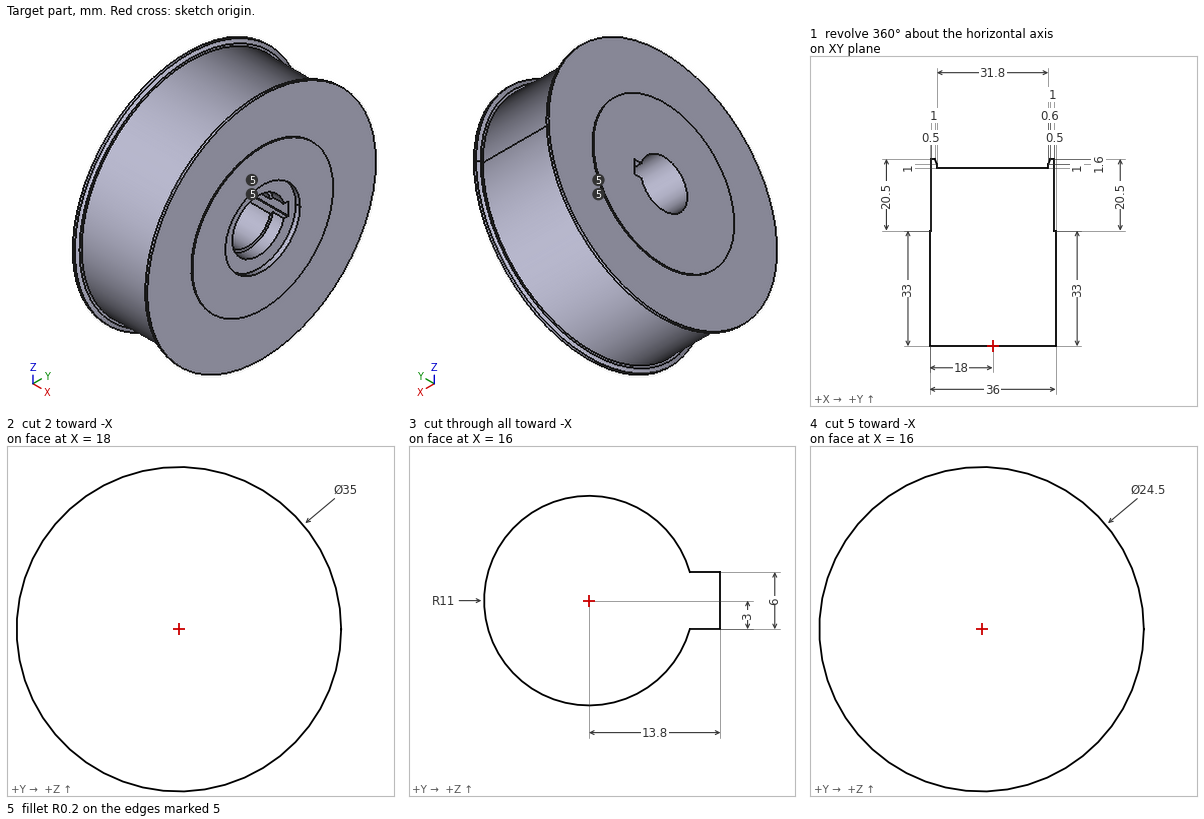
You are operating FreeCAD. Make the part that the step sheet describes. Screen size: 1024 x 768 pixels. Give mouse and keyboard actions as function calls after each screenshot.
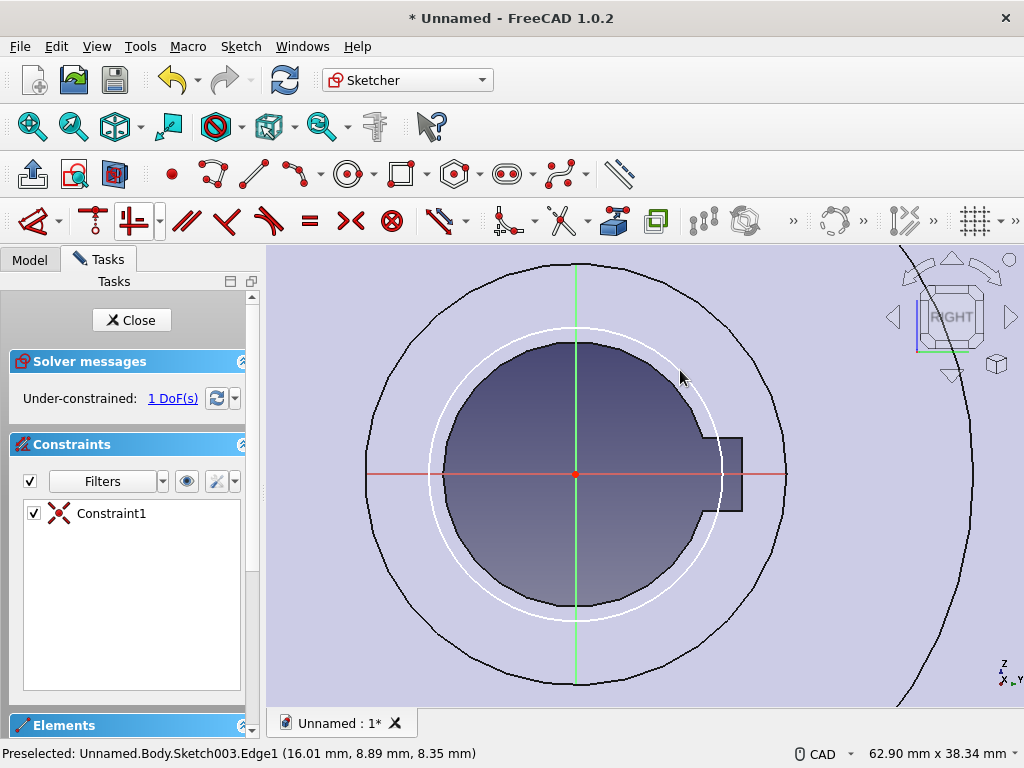
click(32, 222)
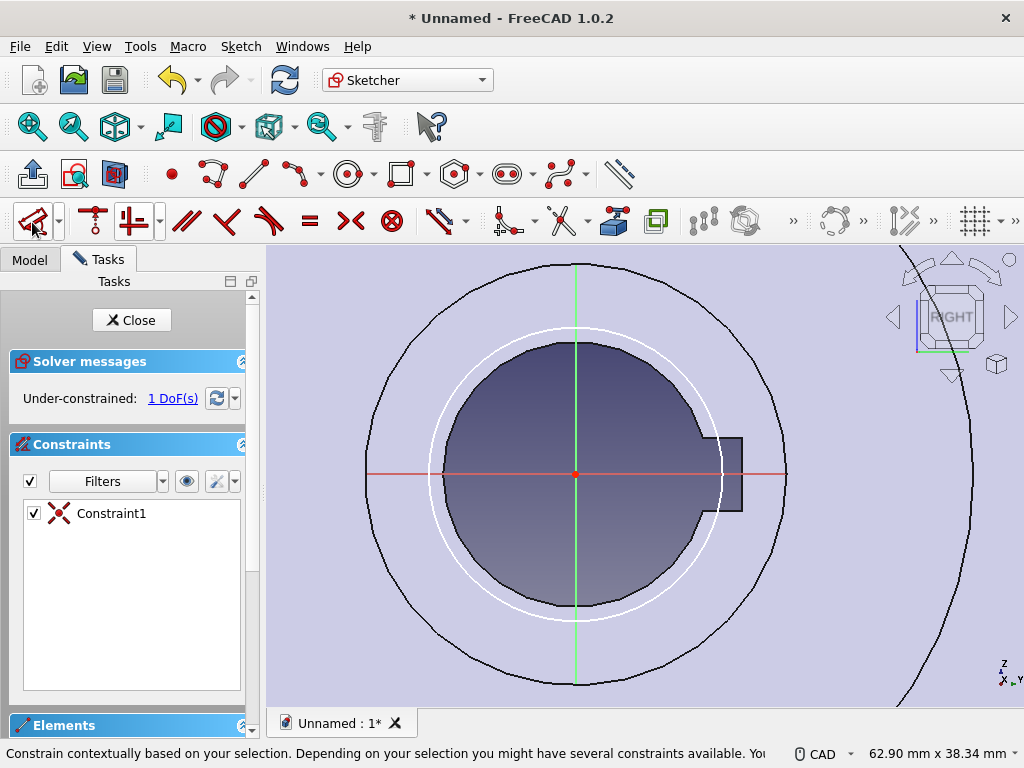
click(679, 370)
click(702, 347)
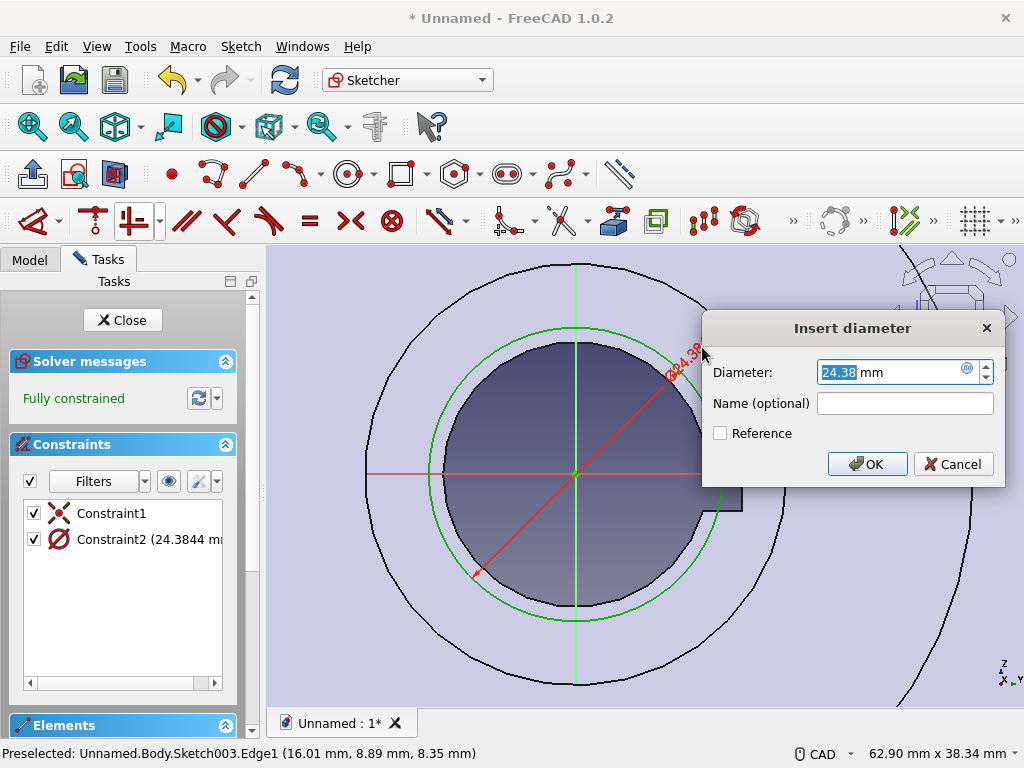
text(24.5)
key(Return)
key(Escape)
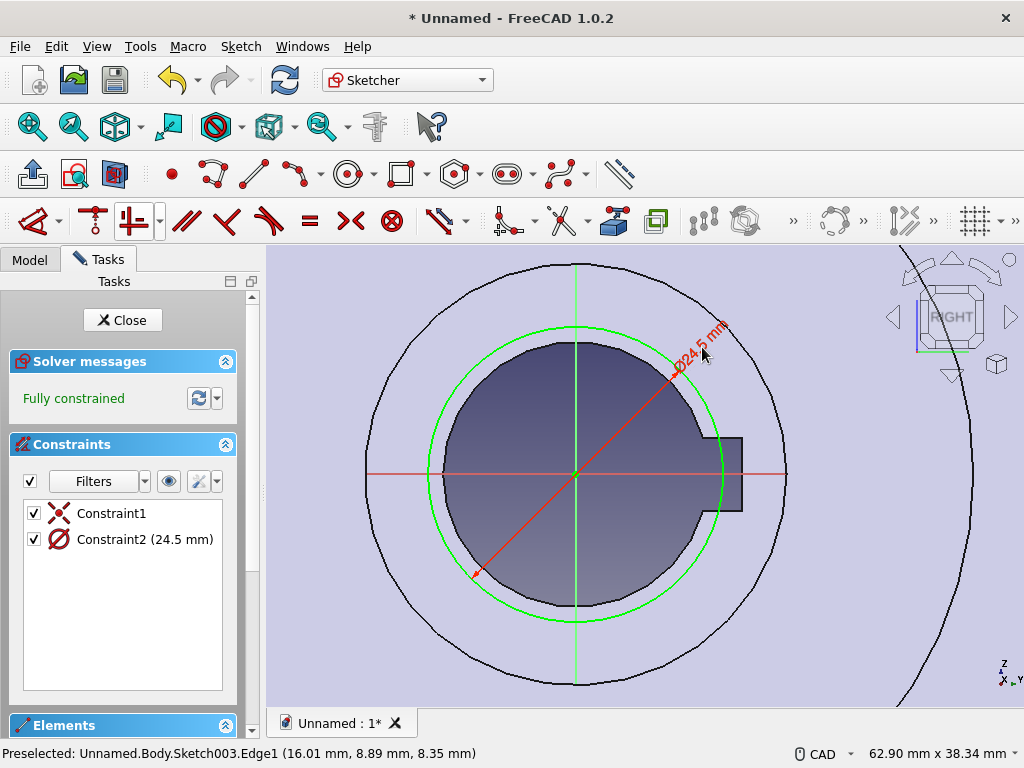
click(123, 320)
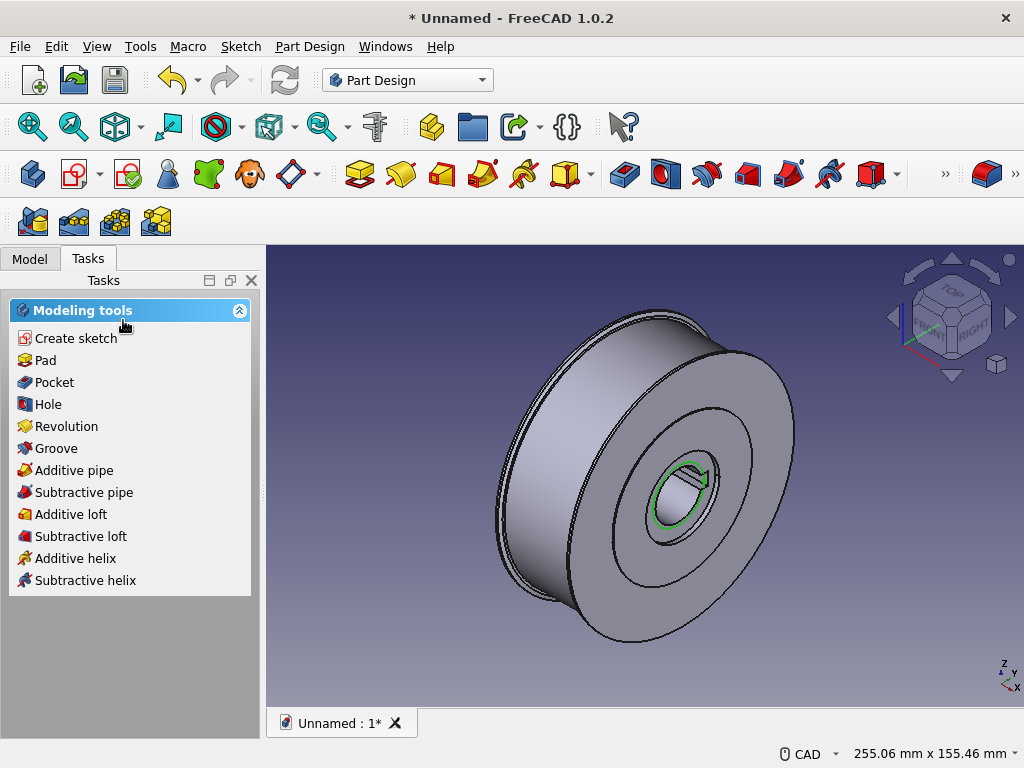
click(625, 174)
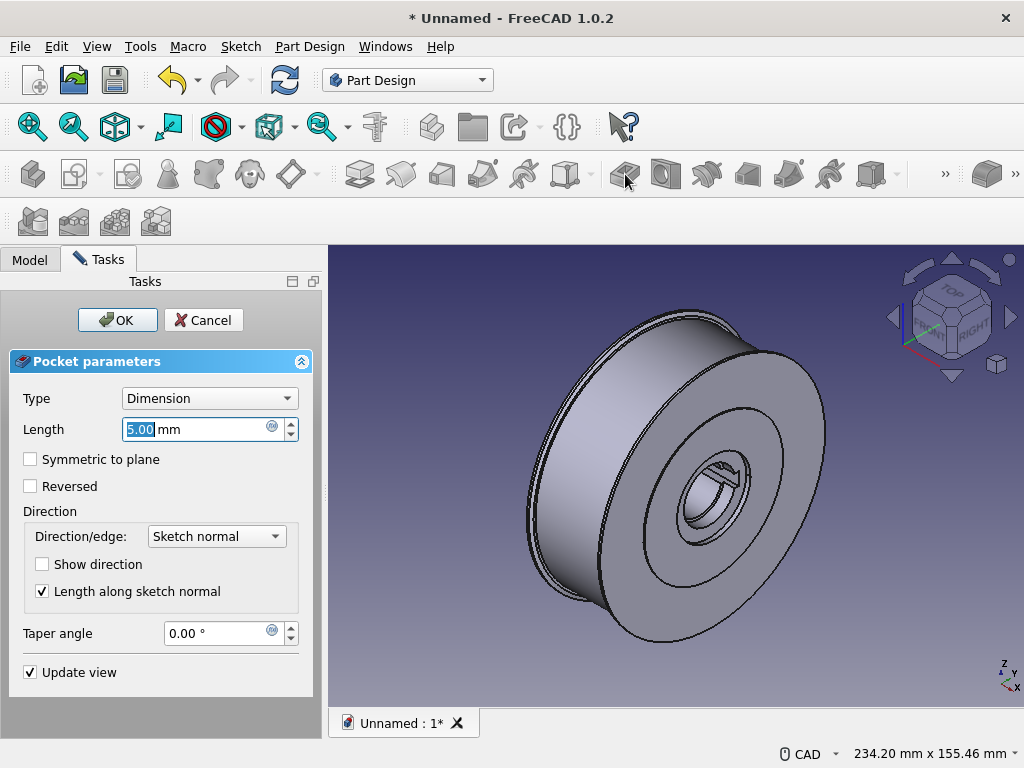
text(5)
key(Tab)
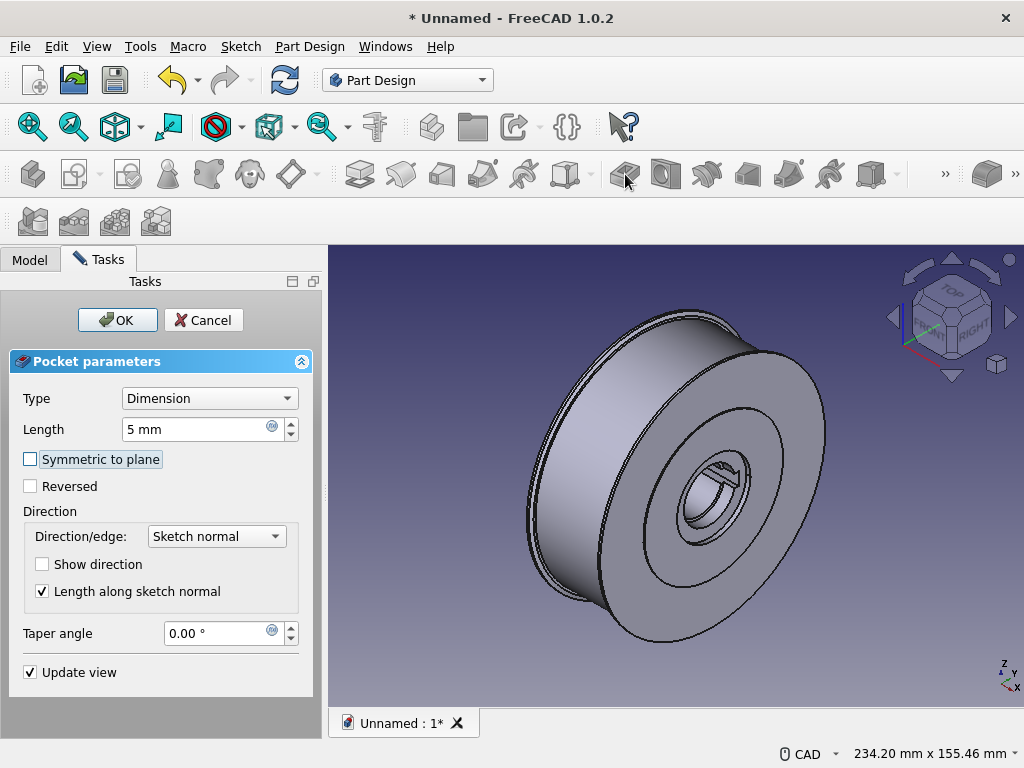
click(118, 320)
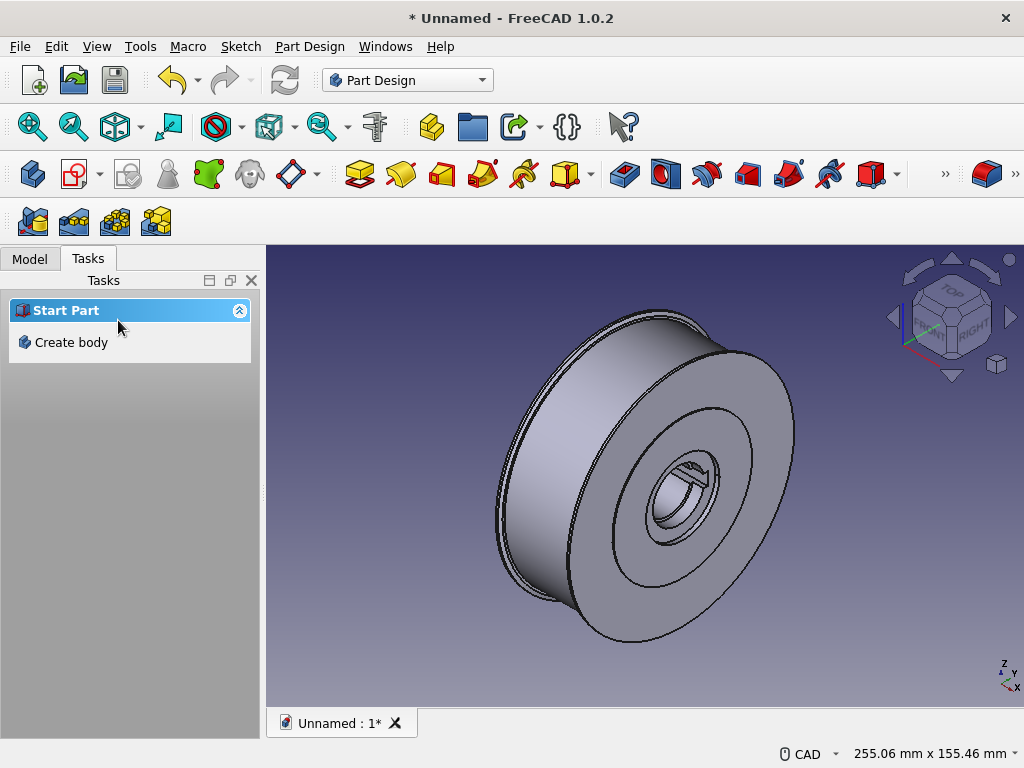
key(2)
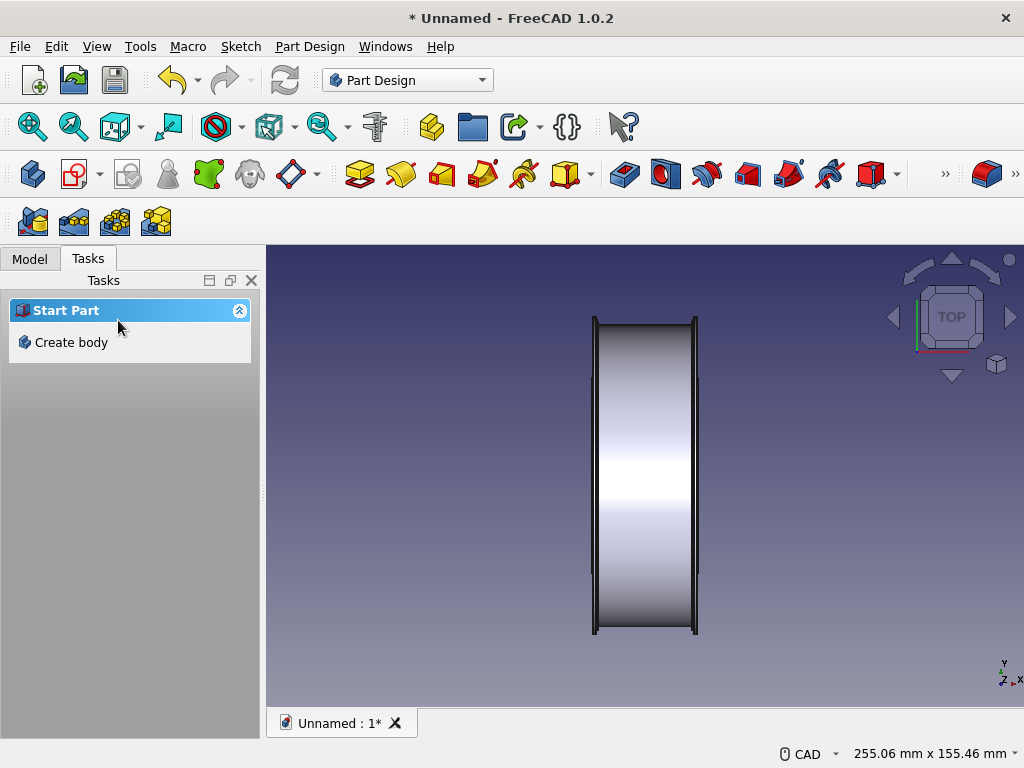
key(0)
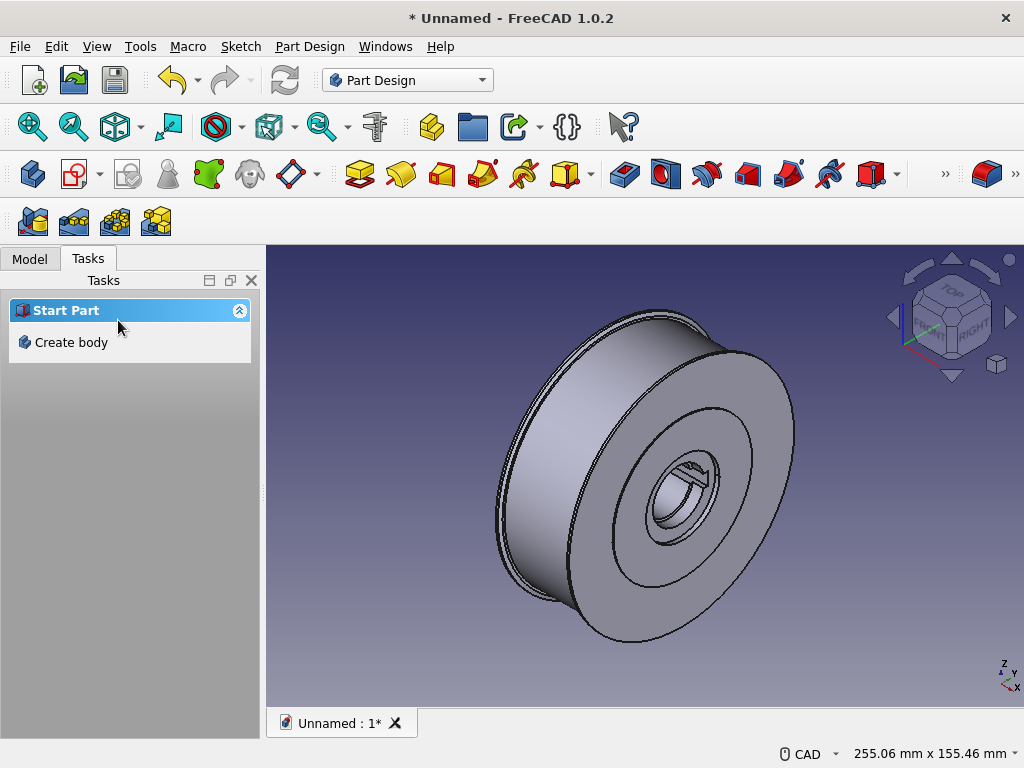
key(1)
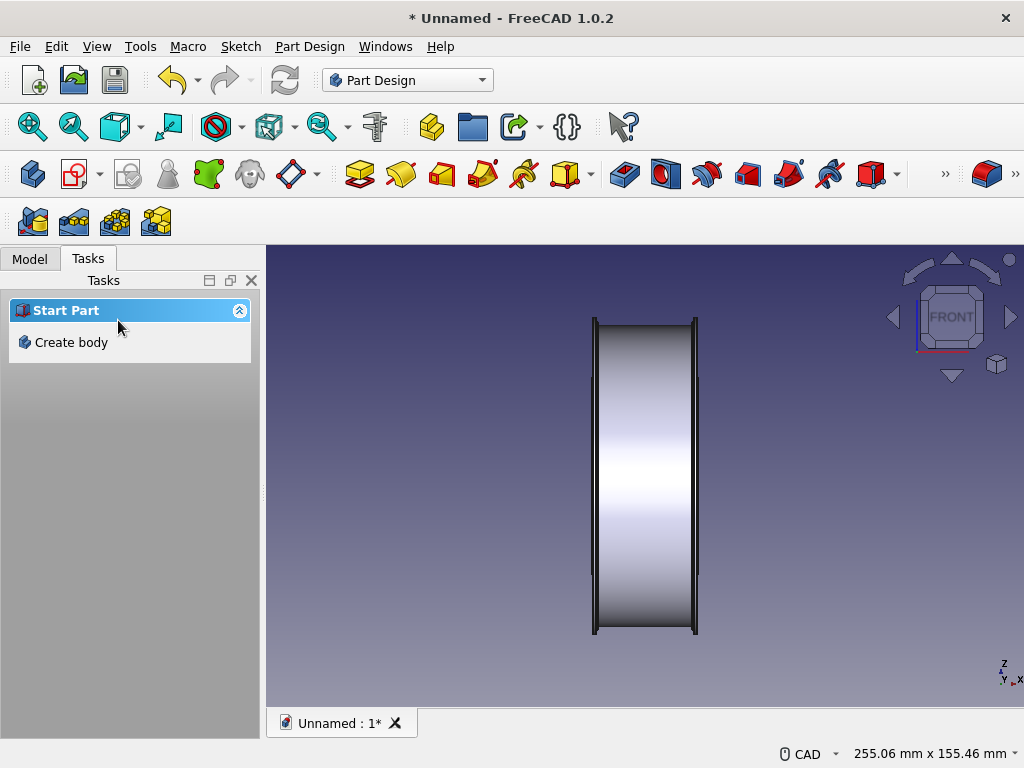
key(3)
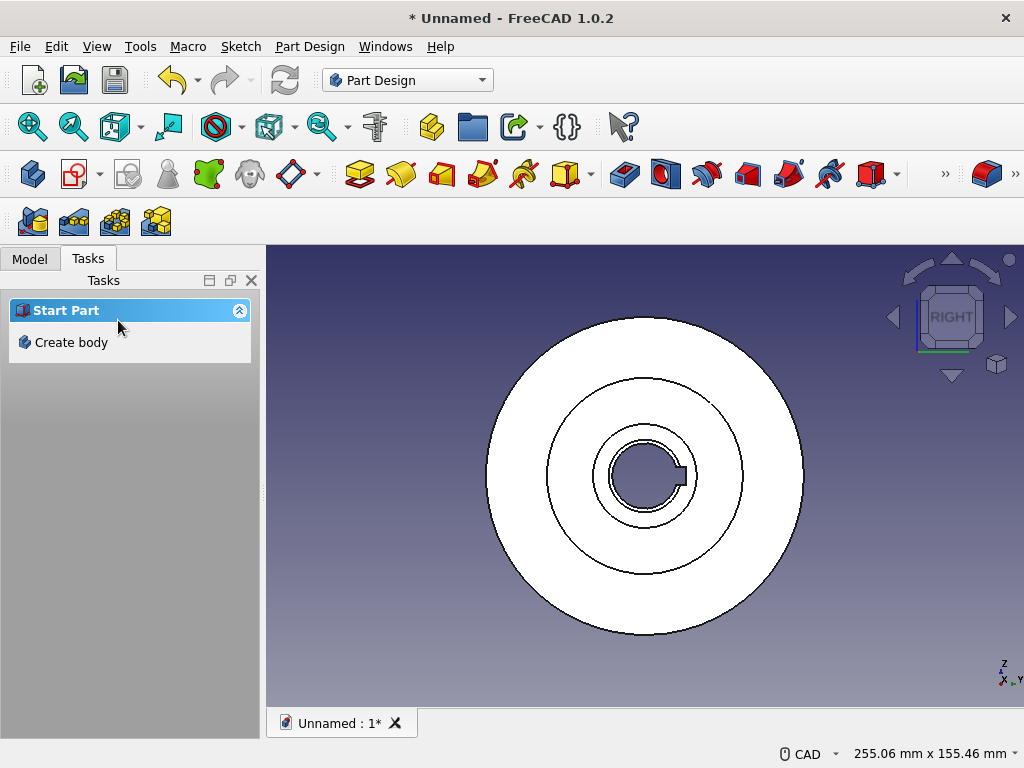
key(5)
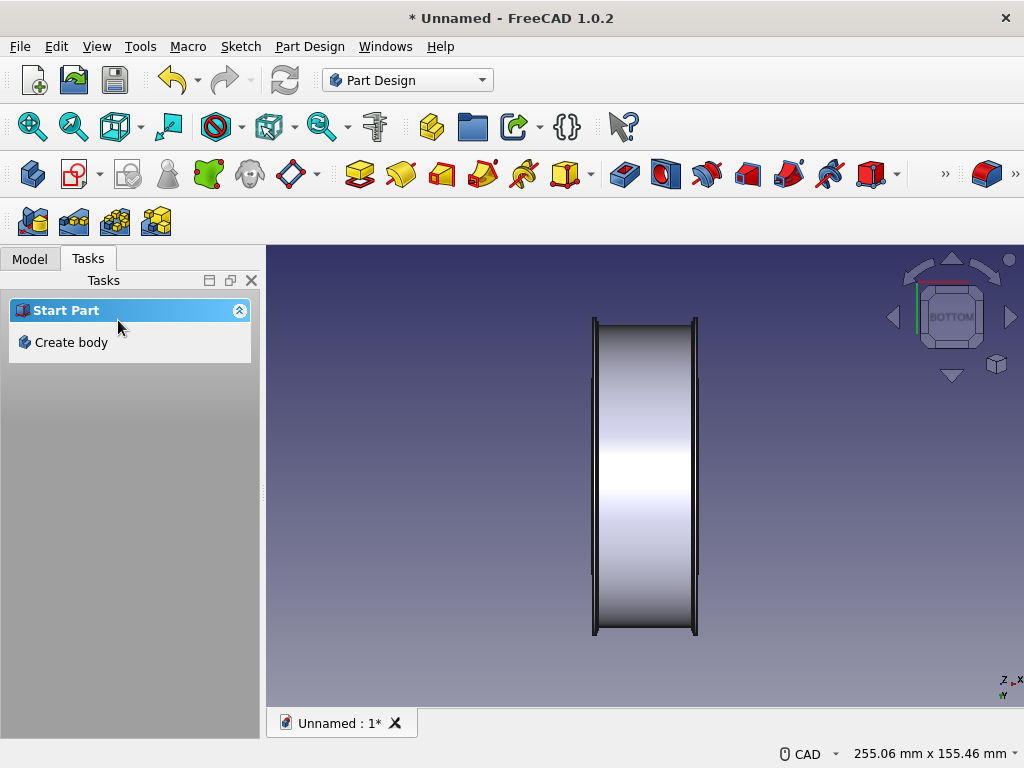
key(4)